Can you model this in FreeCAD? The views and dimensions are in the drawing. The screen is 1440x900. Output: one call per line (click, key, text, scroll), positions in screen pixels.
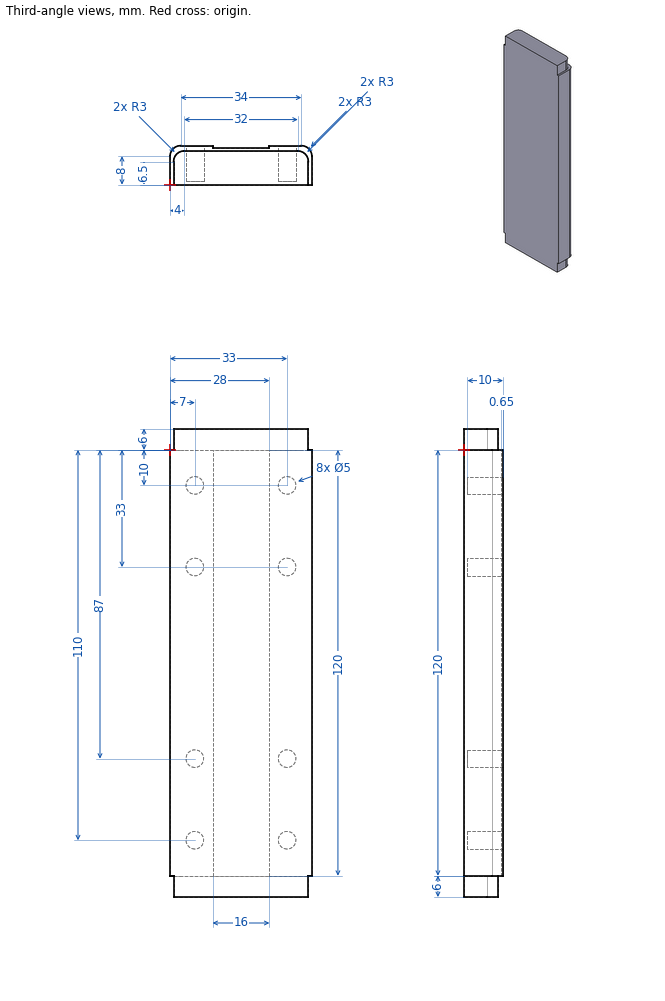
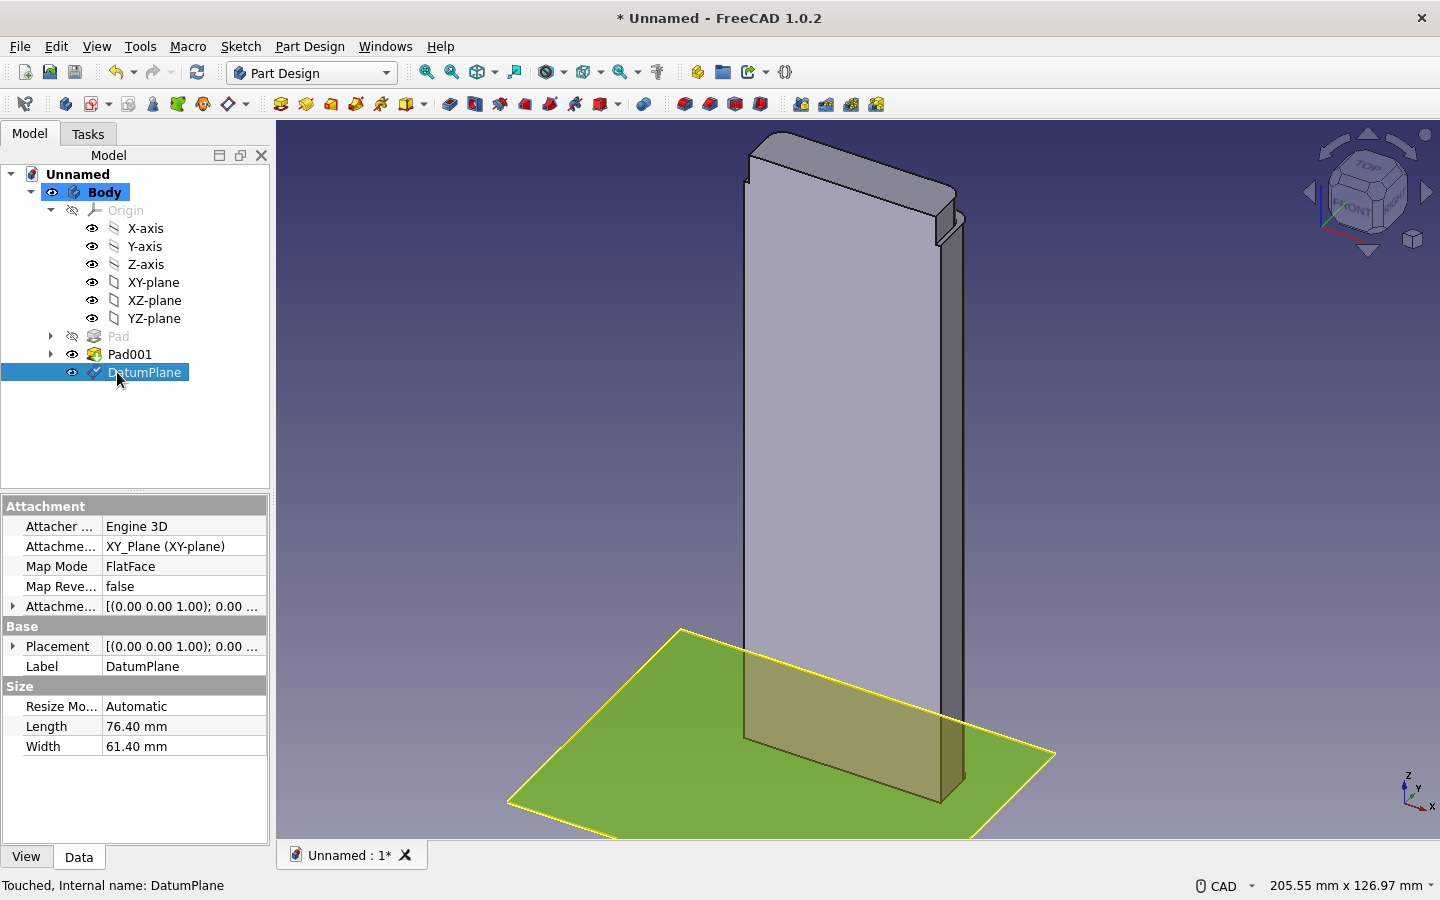
click(90, 104)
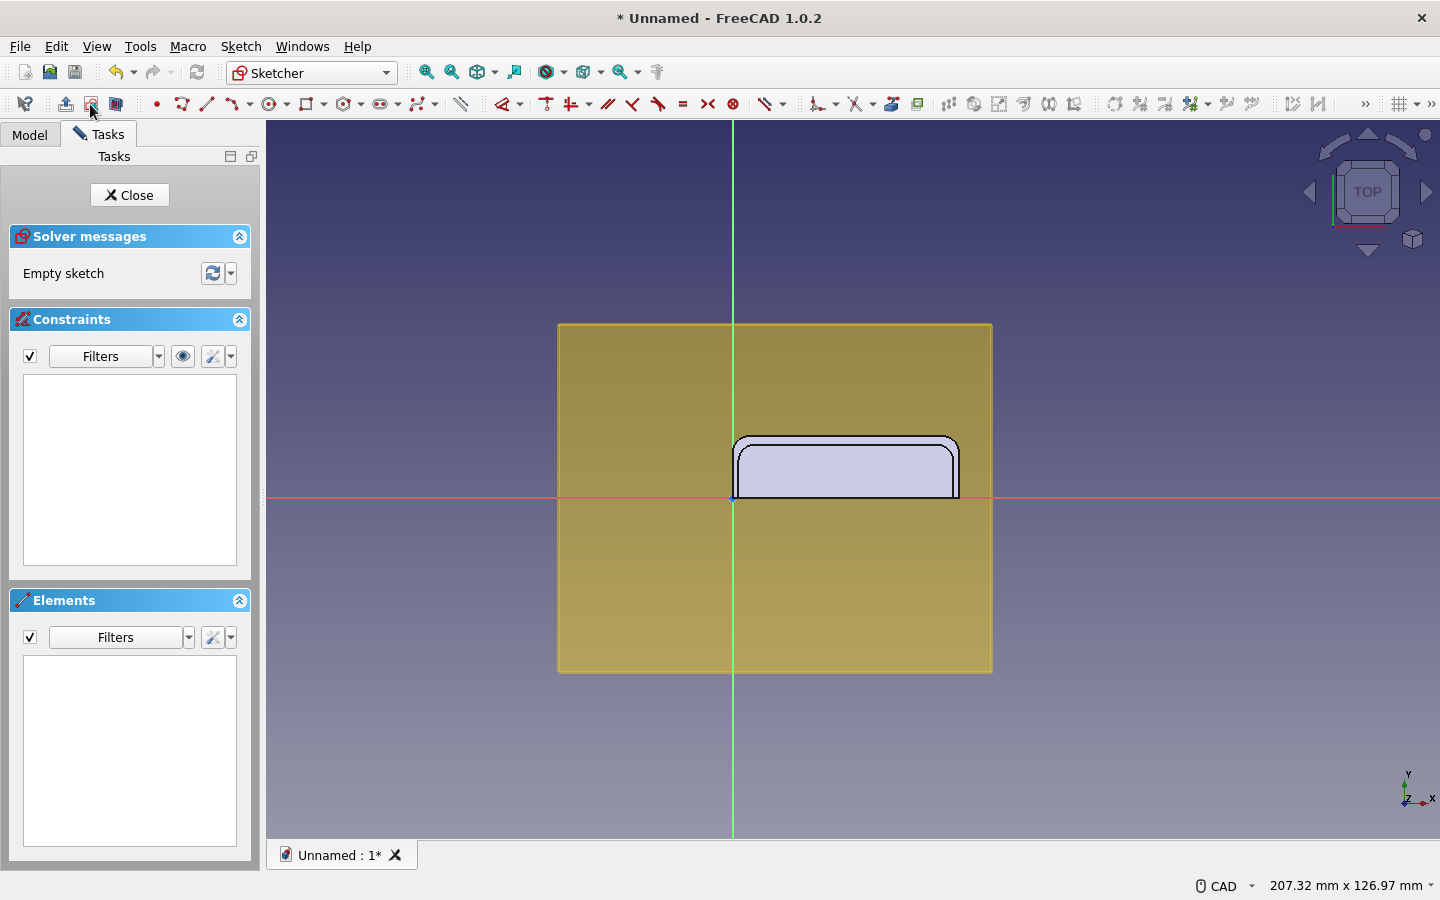
click(116, 104)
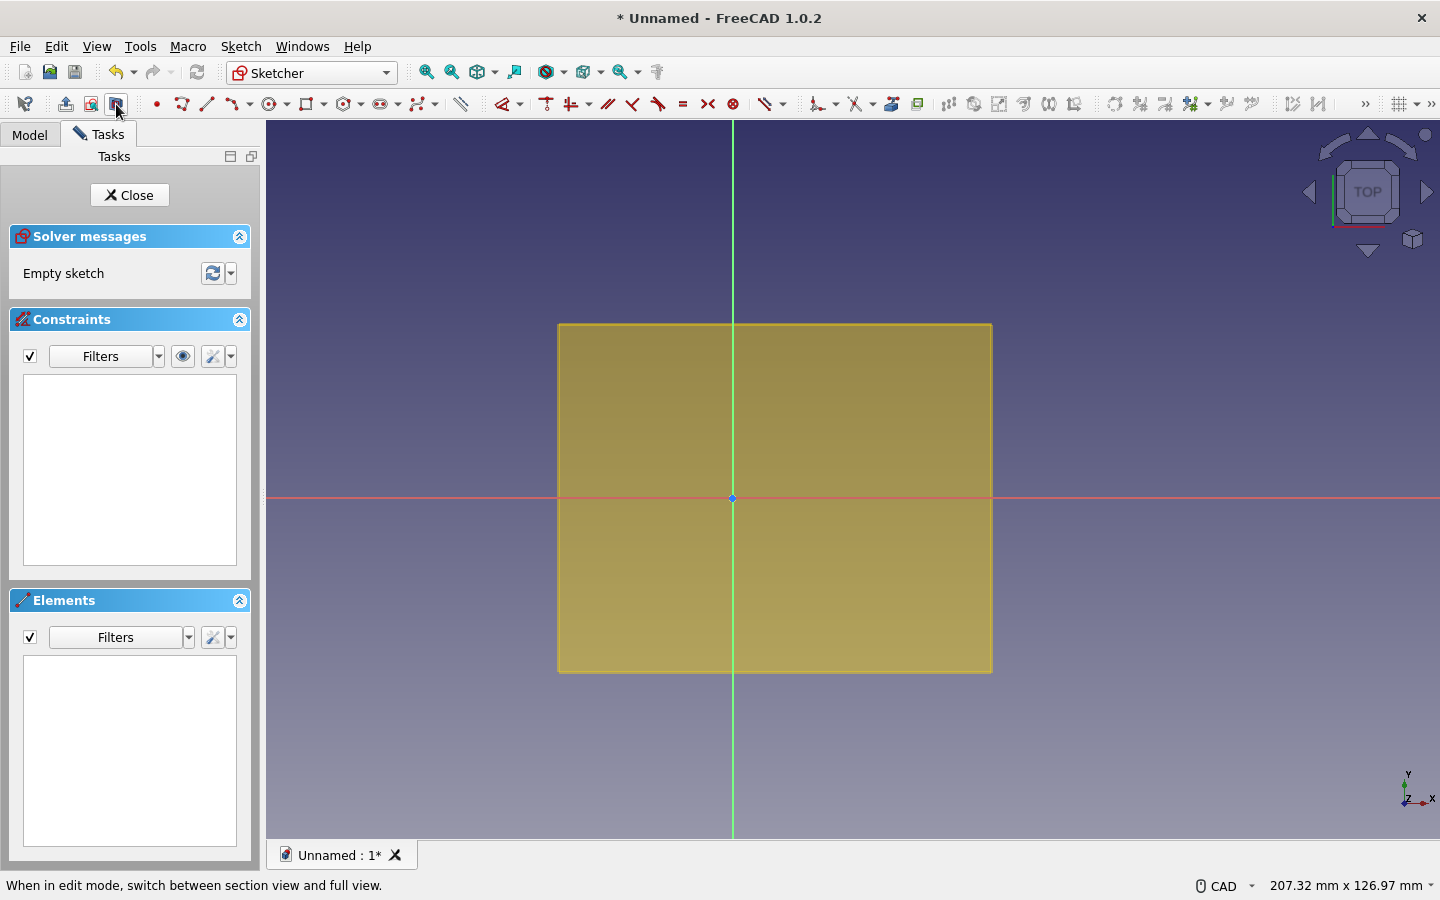
scroll(868, 468, up, 6)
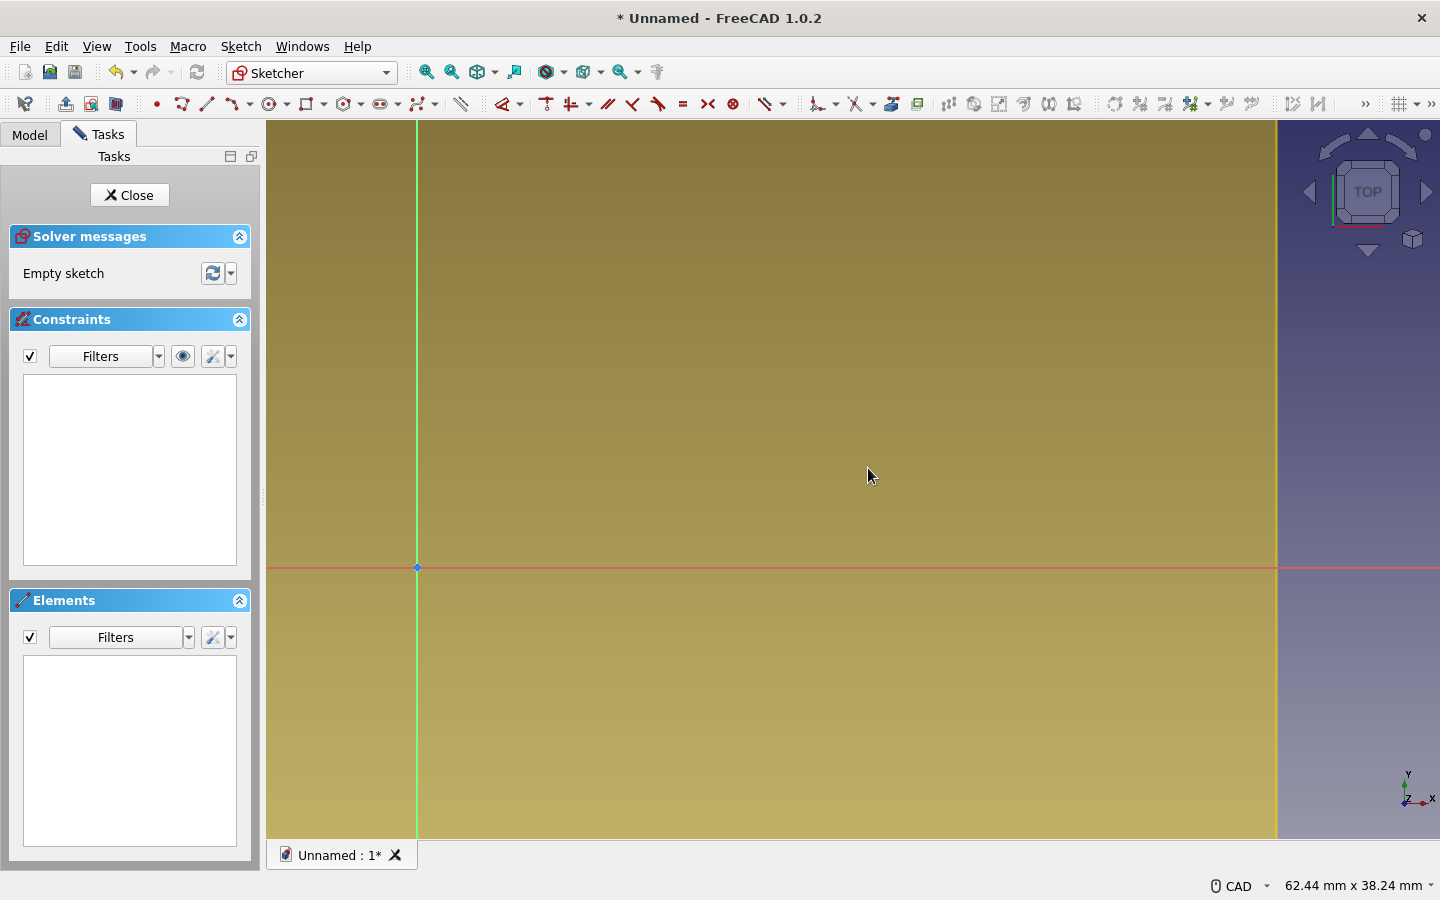
click(207, 104)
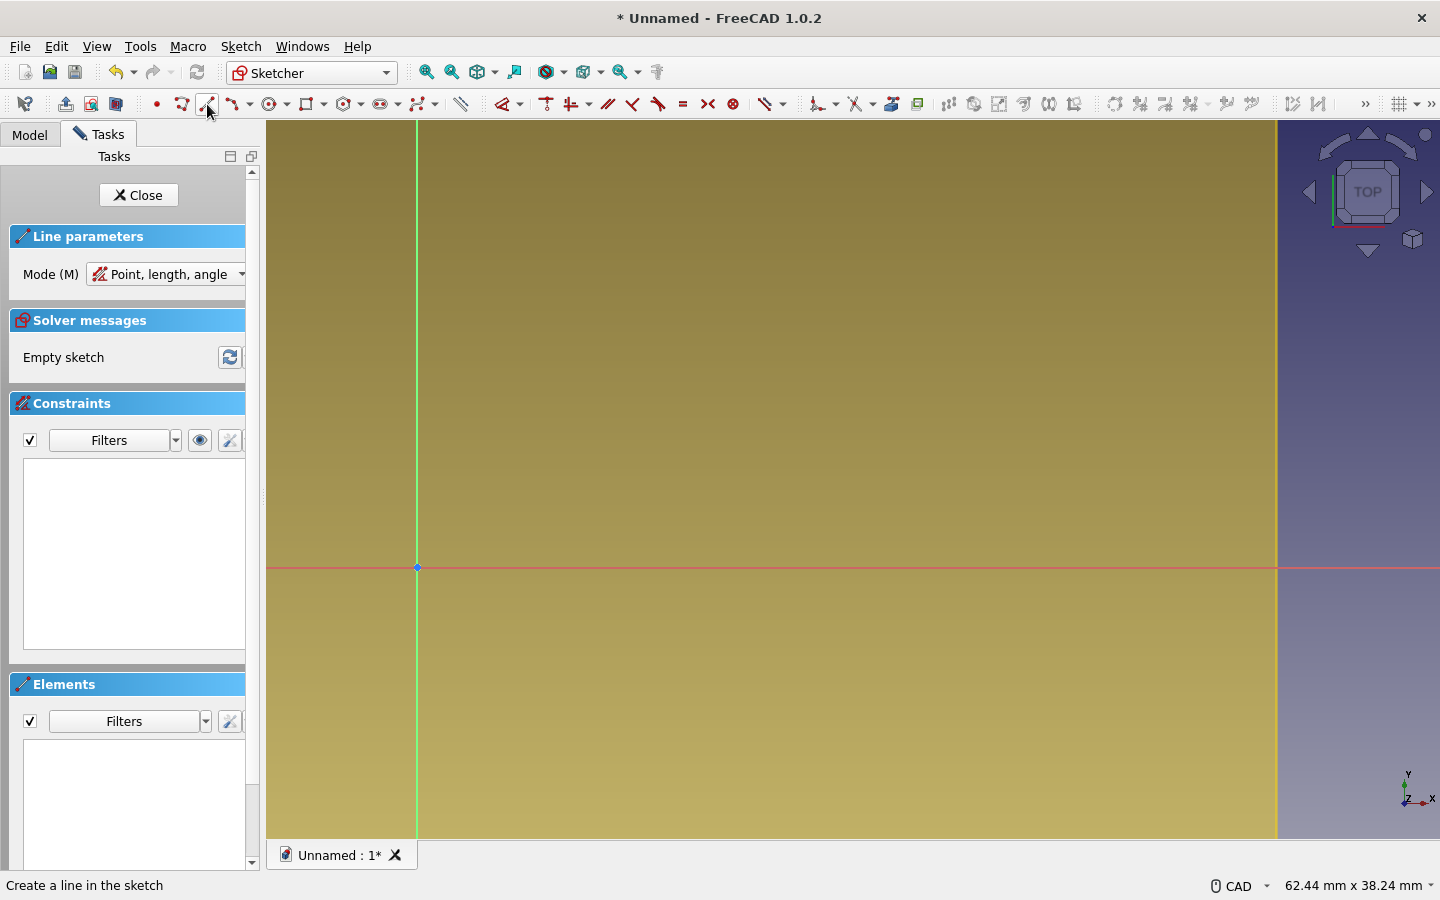
click(493, 389)
click(1094, 389)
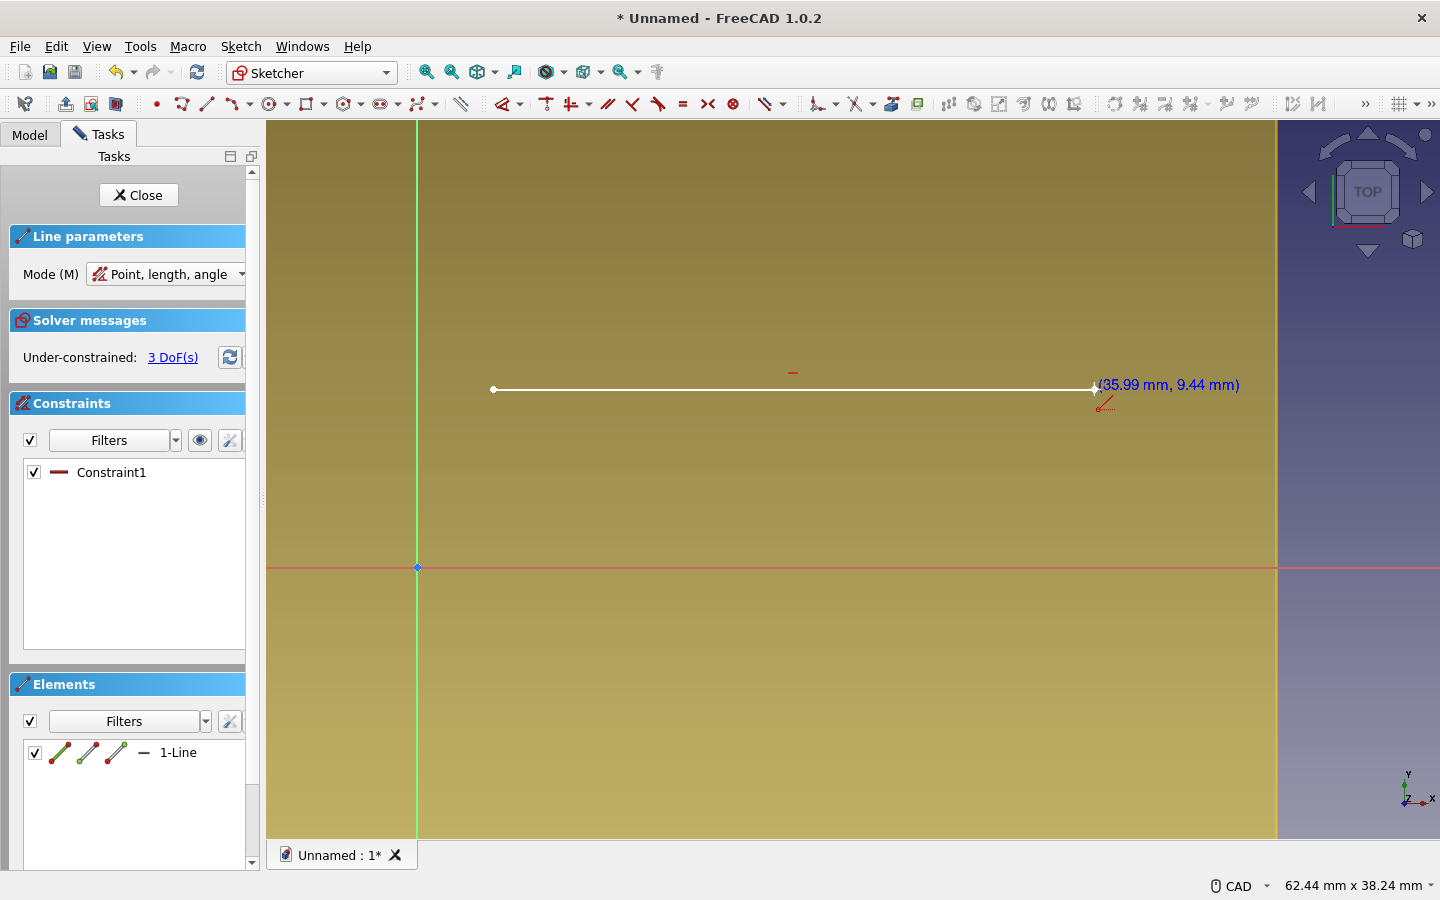
key(g)
key(m)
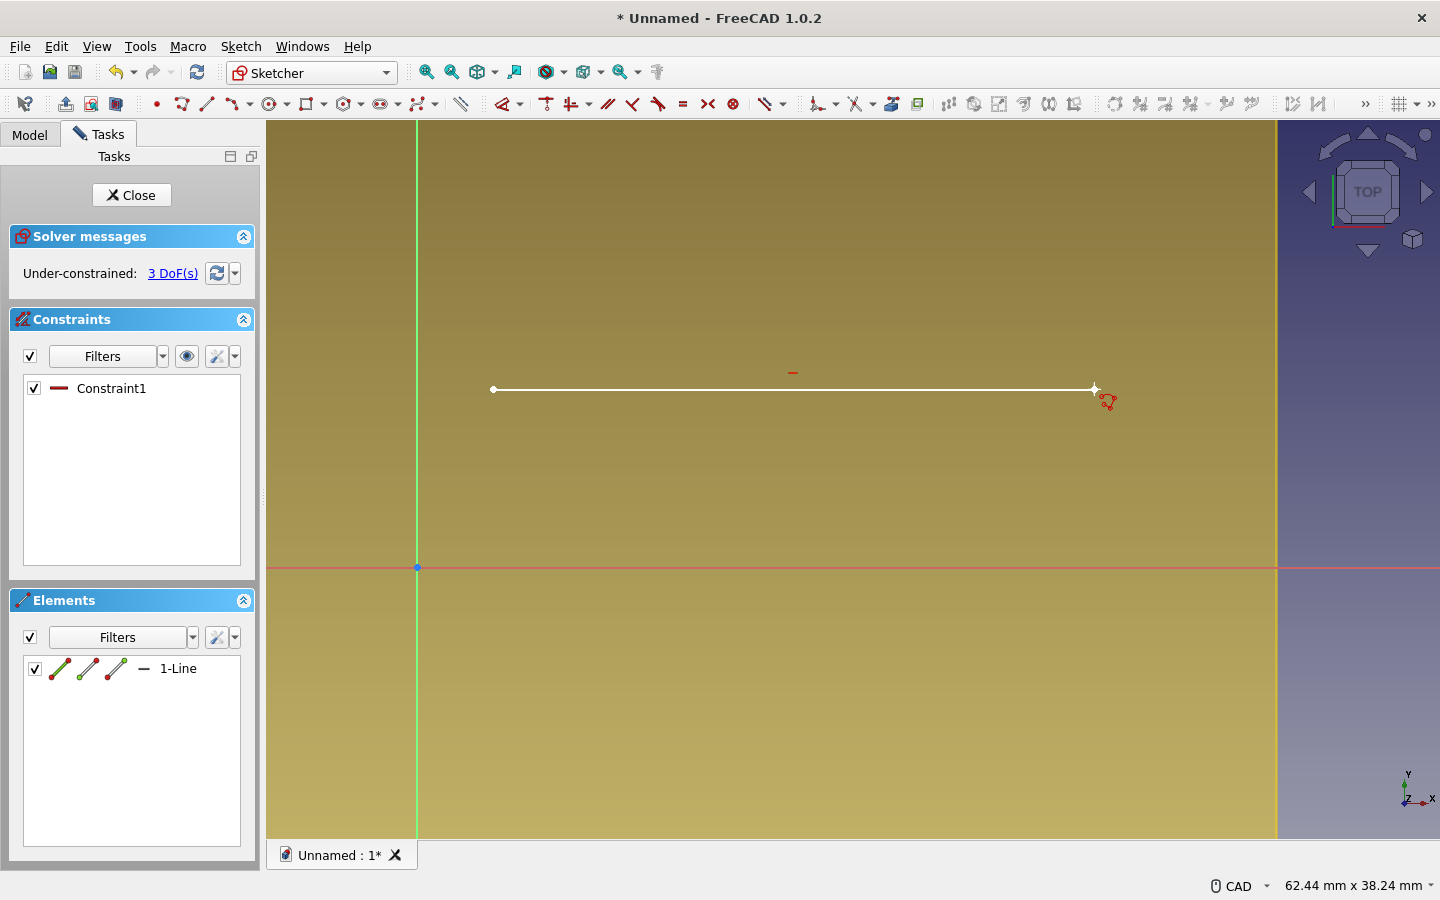
click(1151, 445)
click(1151, 568)
click(436, 559)
click(436, 445)
right_click(436, 445)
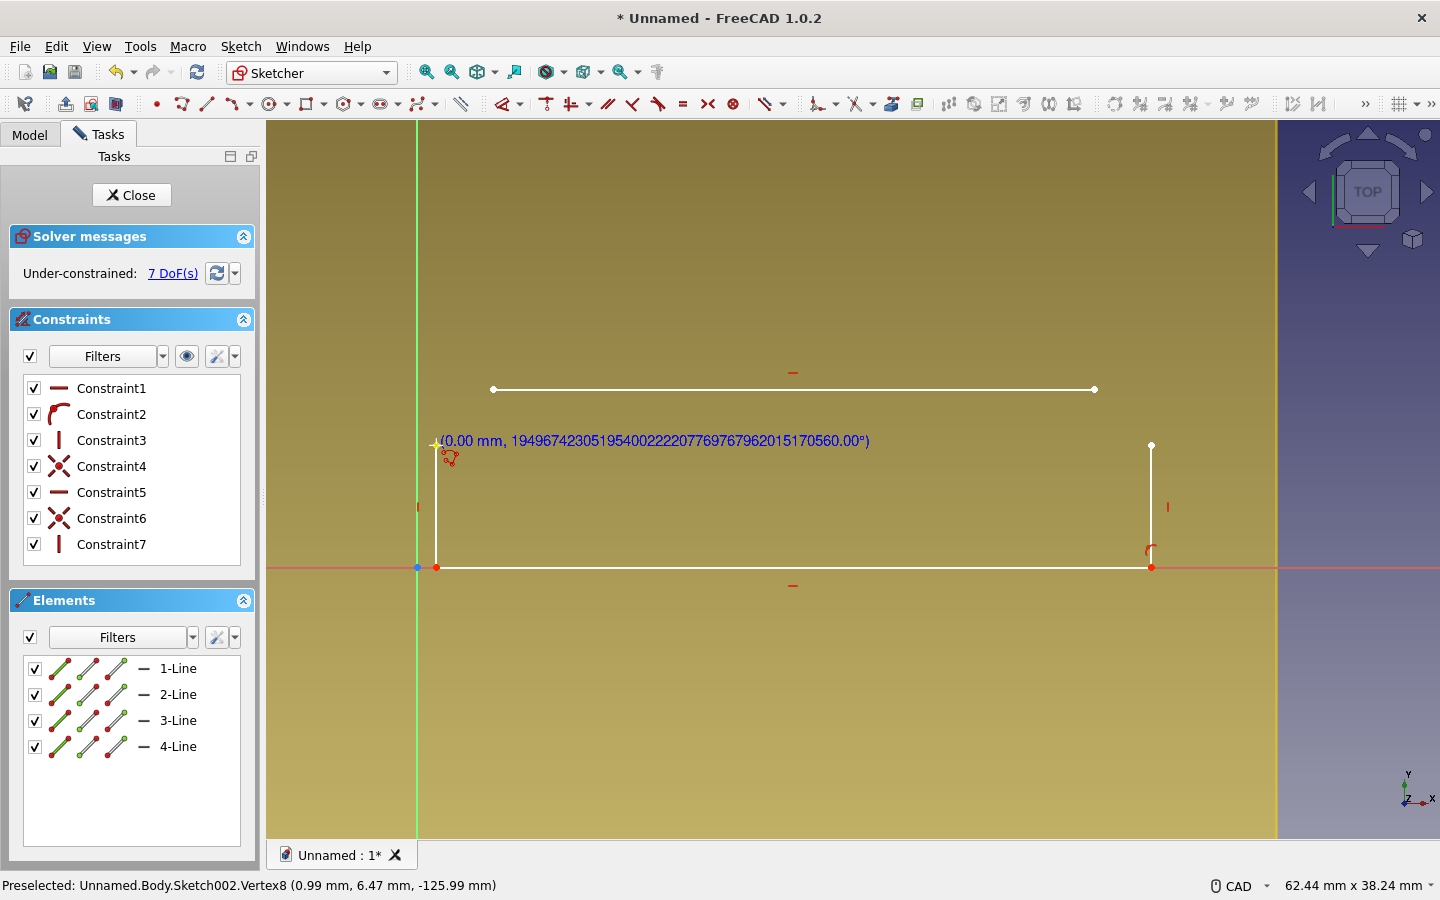
click(232, 104)